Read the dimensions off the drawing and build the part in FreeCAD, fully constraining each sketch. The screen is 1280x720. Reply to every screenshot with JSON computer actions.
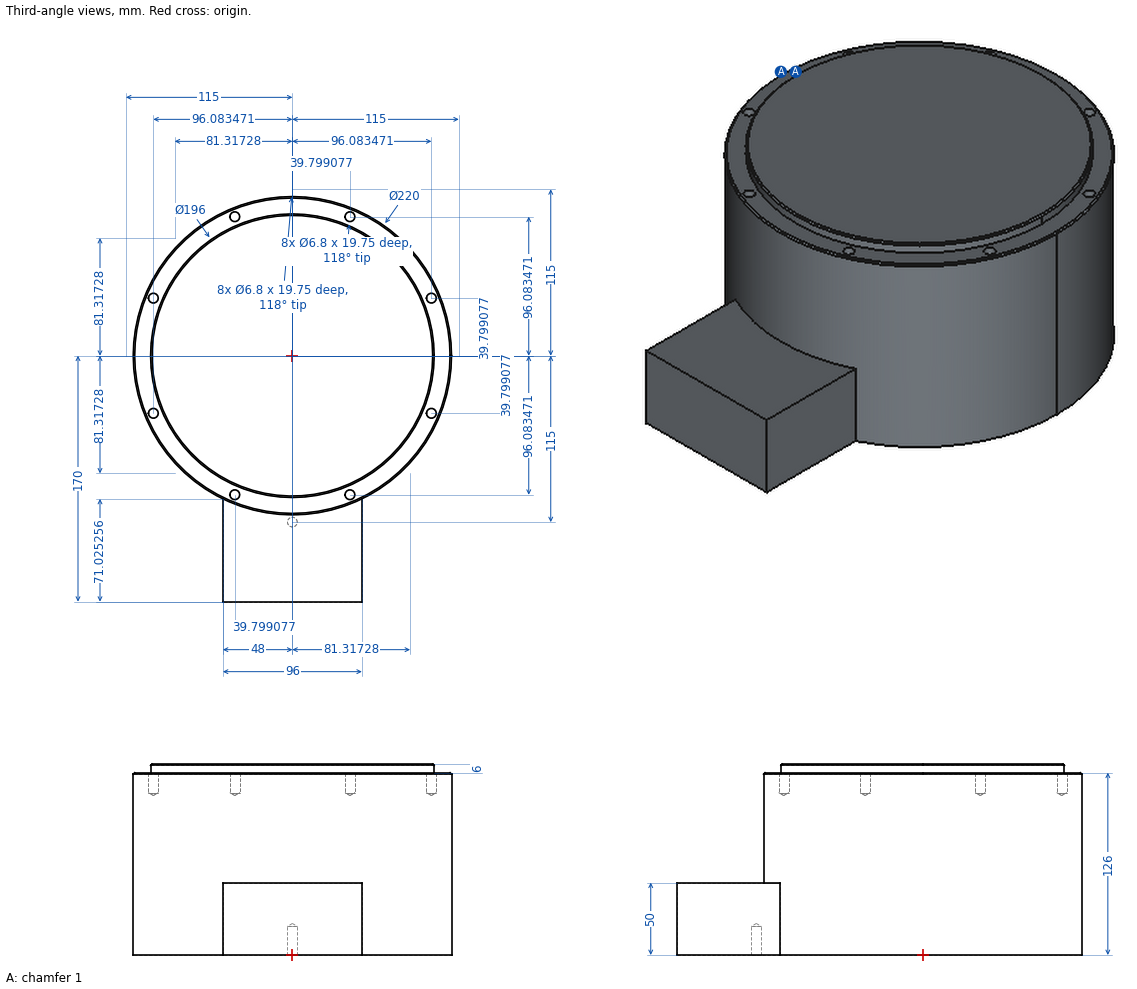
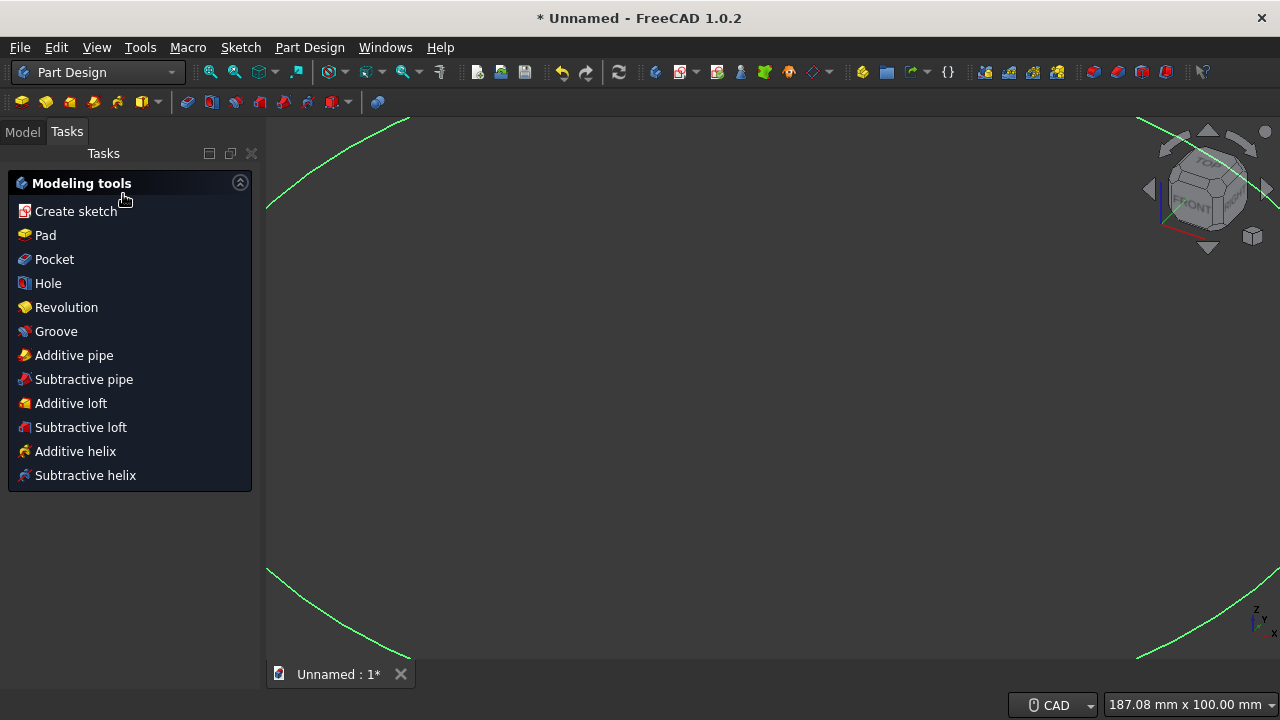
{"action": "left_click", "coordinate": [22, 102]}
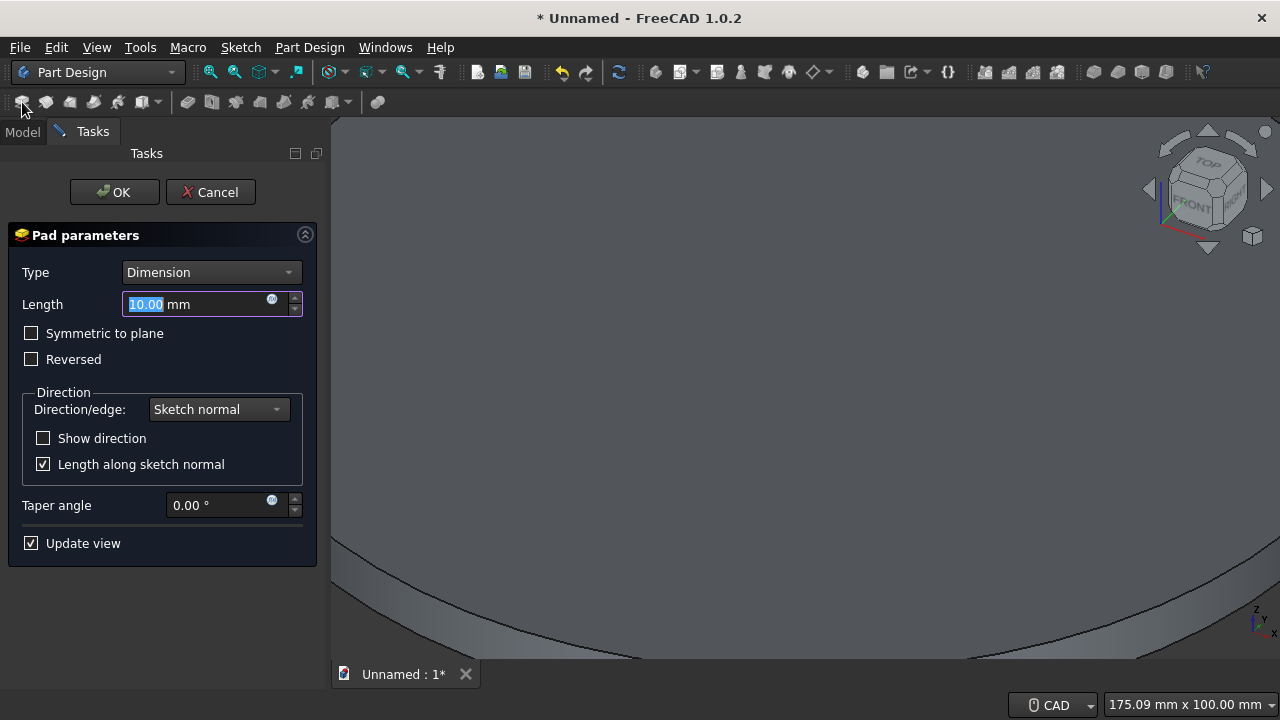
{"action": "type", "text": "126"}
{"action": "key", "text": "Tab"}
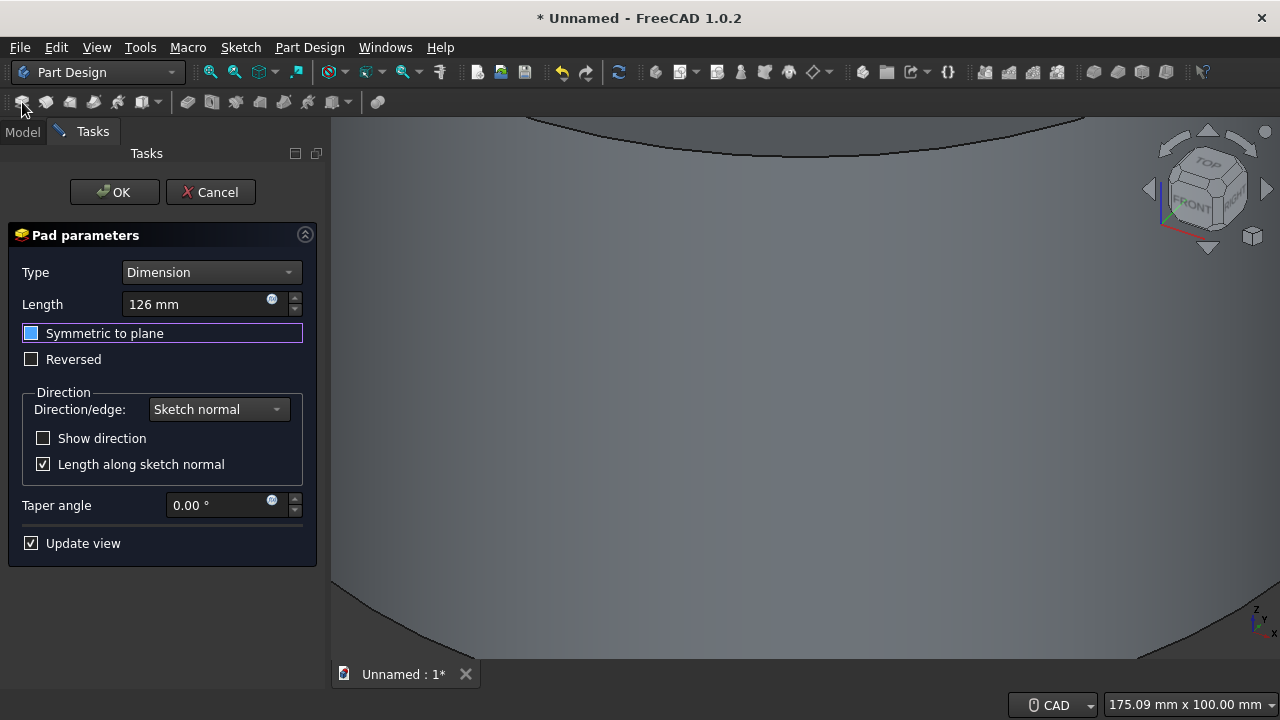
{"action": "left_click", "coordinate": [115, 192]}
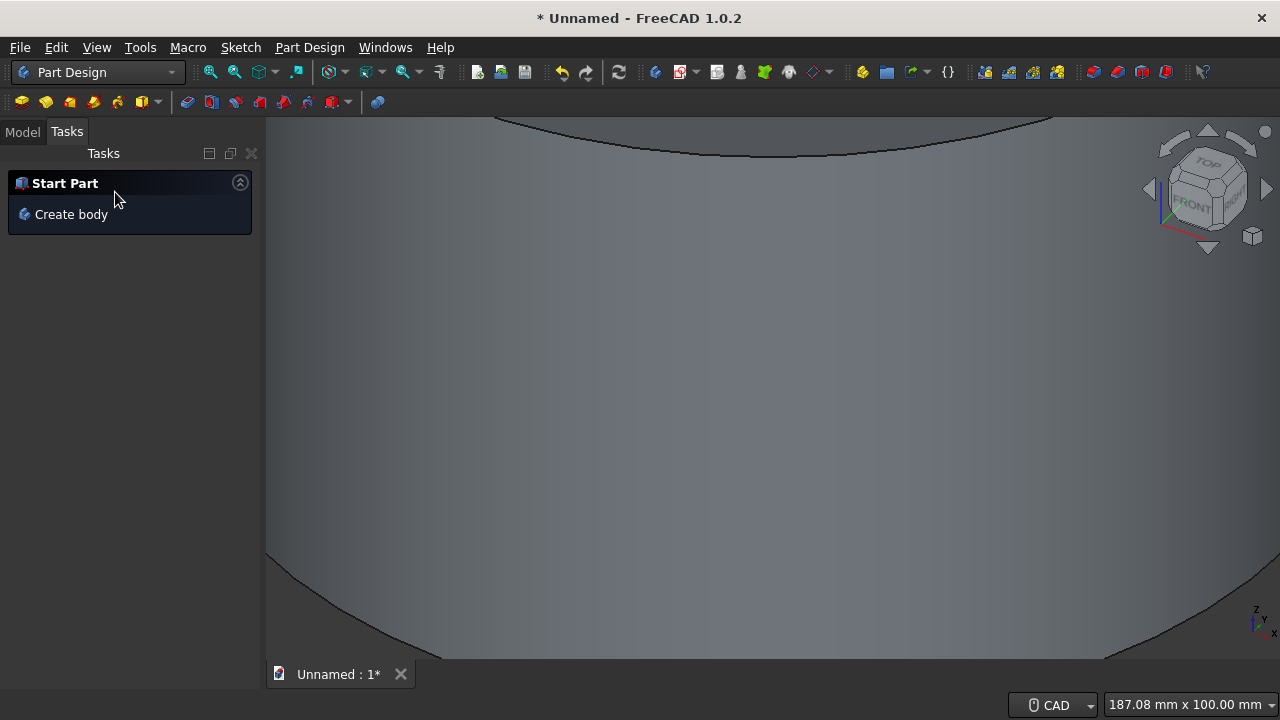
{"action": "left_click", "coordinate": [212, 72]}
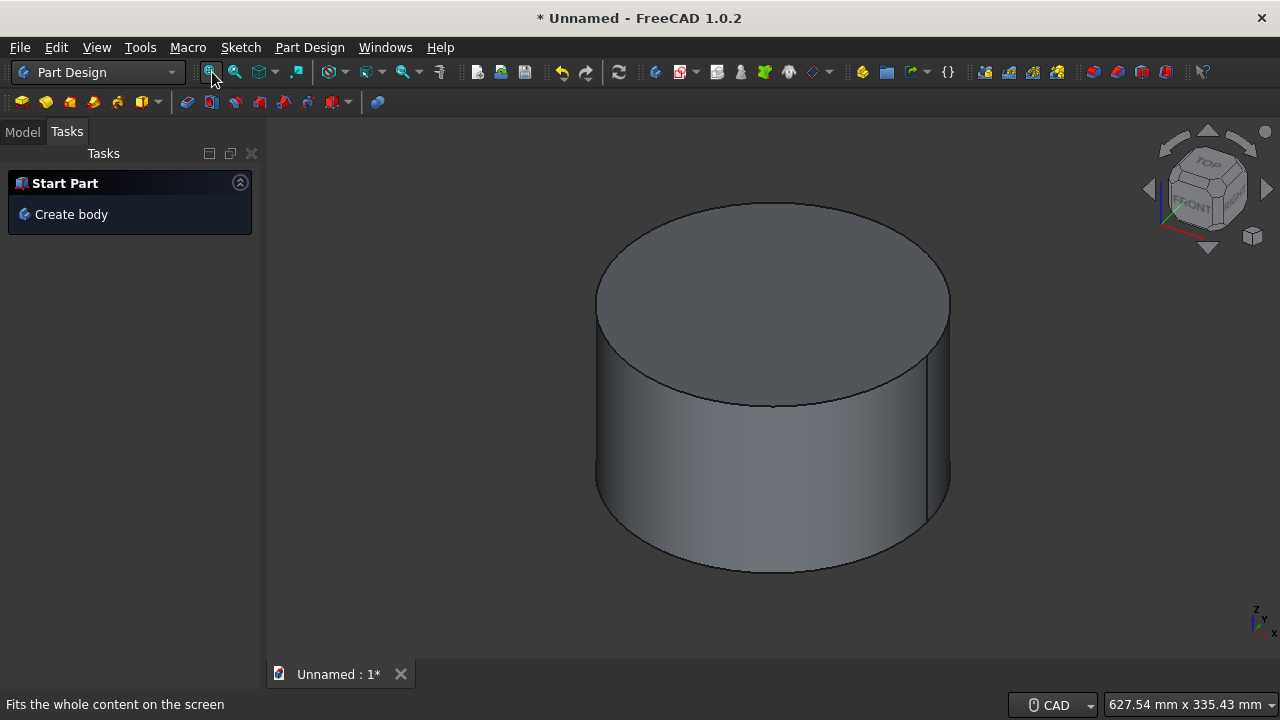
{"action": "left_click", "coordinate": [773, 304]}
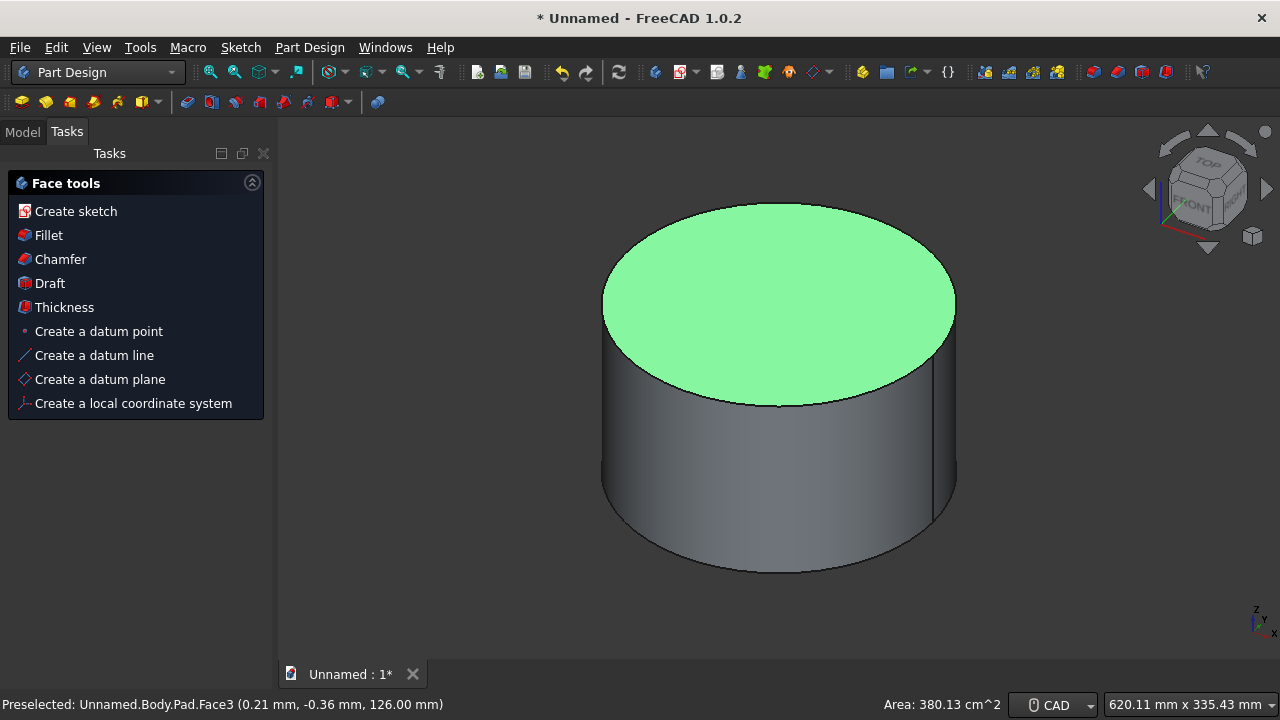
{"action": "left_click", "coordinate": [680, 72]}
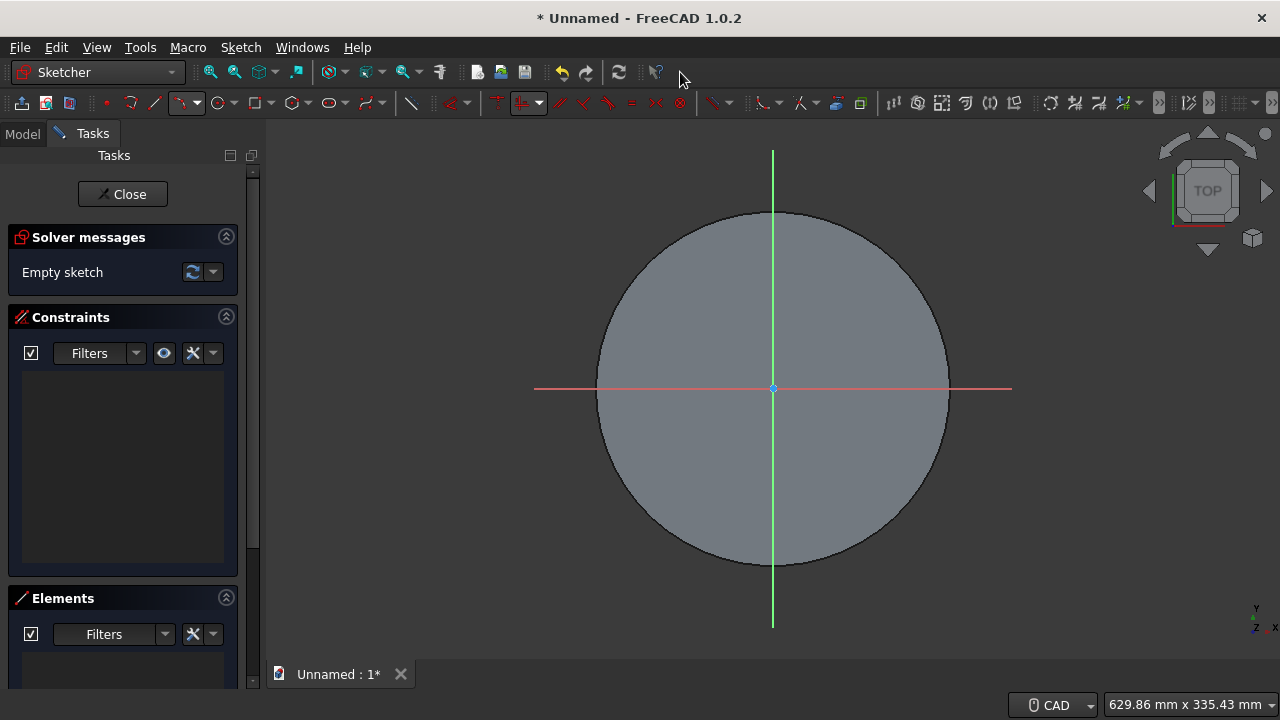
{"action": "left_click", "coordinate": [218, 104]}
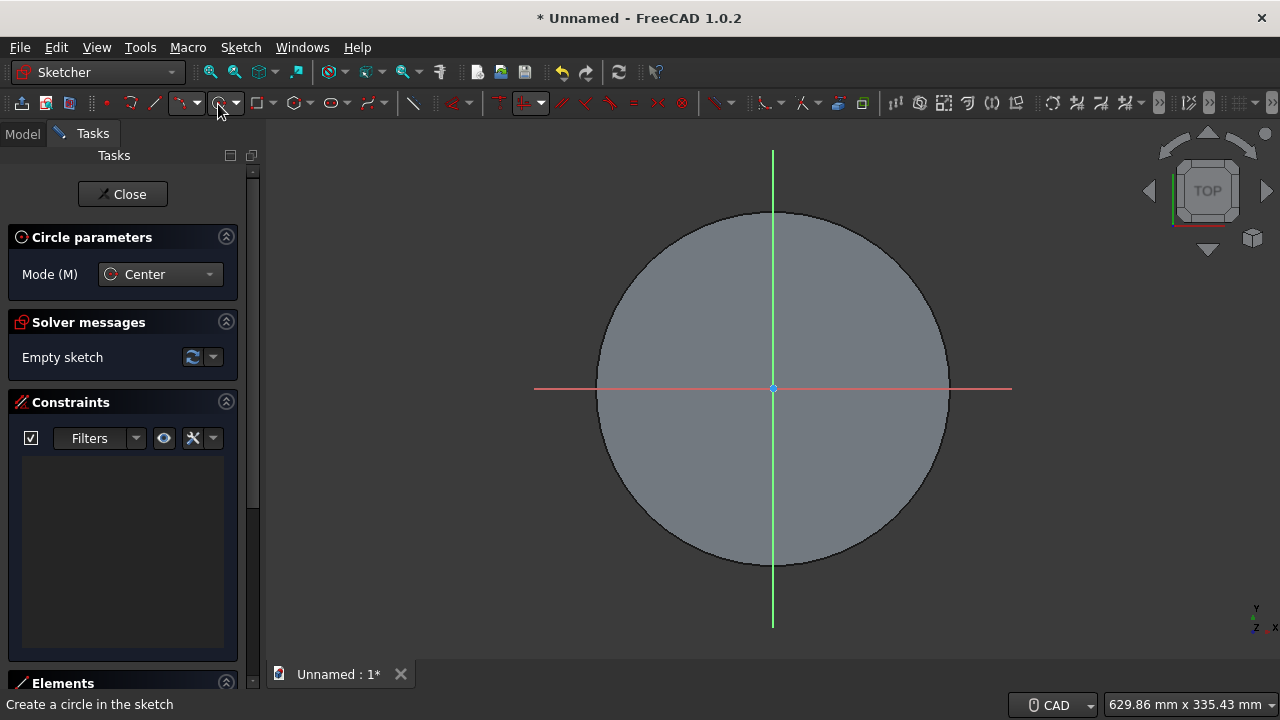
{"action": "left_click", "coordinate": [773, 389]}
{"action": "left_click", "coordinate": [885, 277]}
{"action": "key", "text": "Escape"}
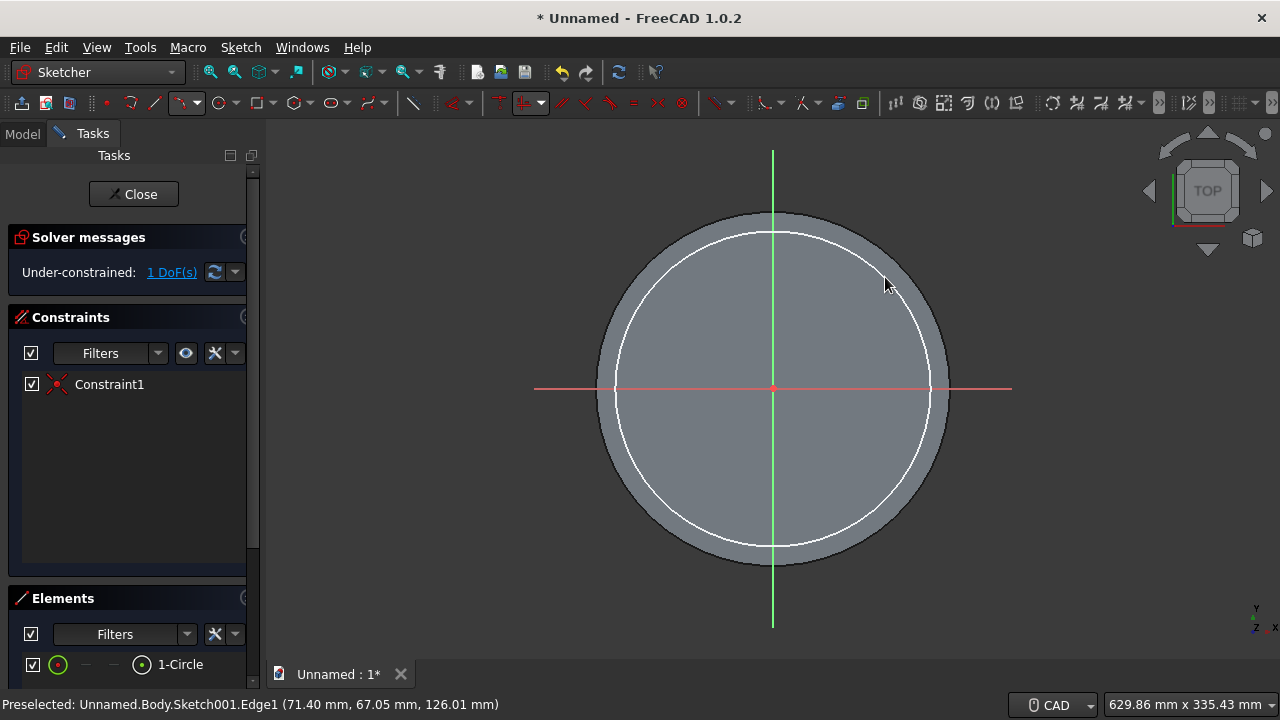
{"action": "left_click", "coordinate": [452, 104]}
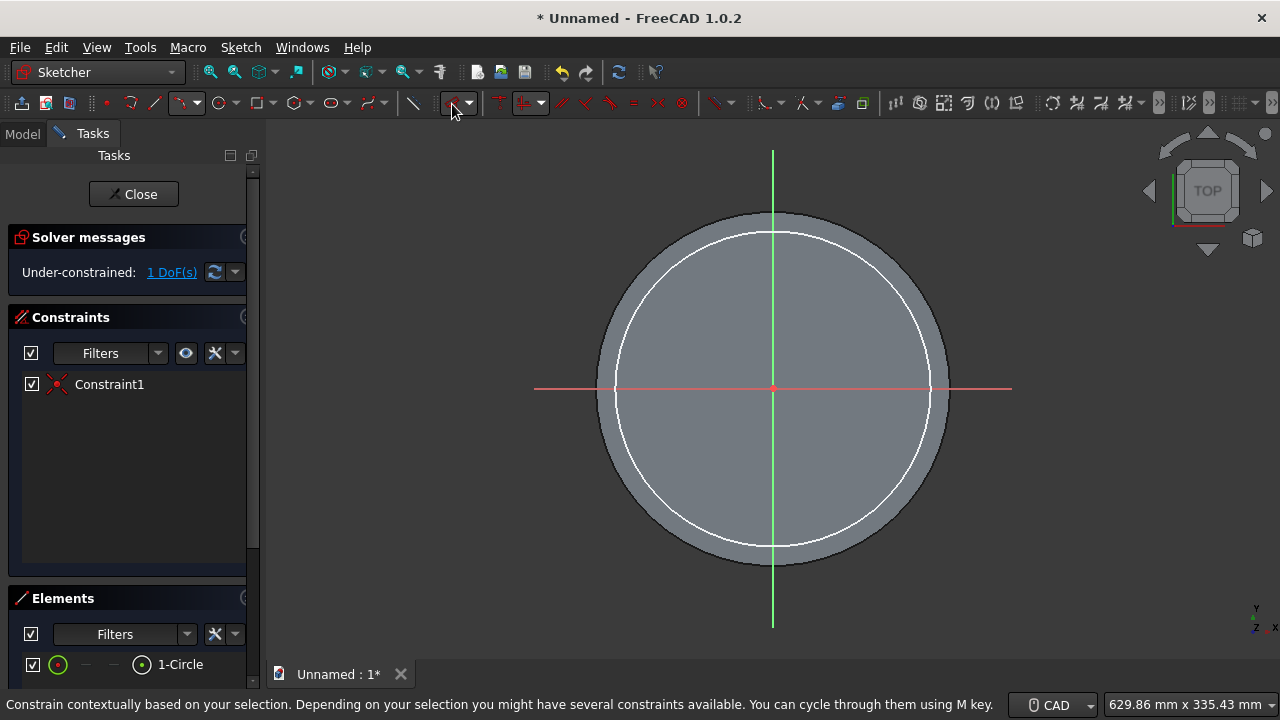
{"action": "left_click", "coordinate": [884, 277]}
{"action": "left_click", "coordinate": [907, 254]}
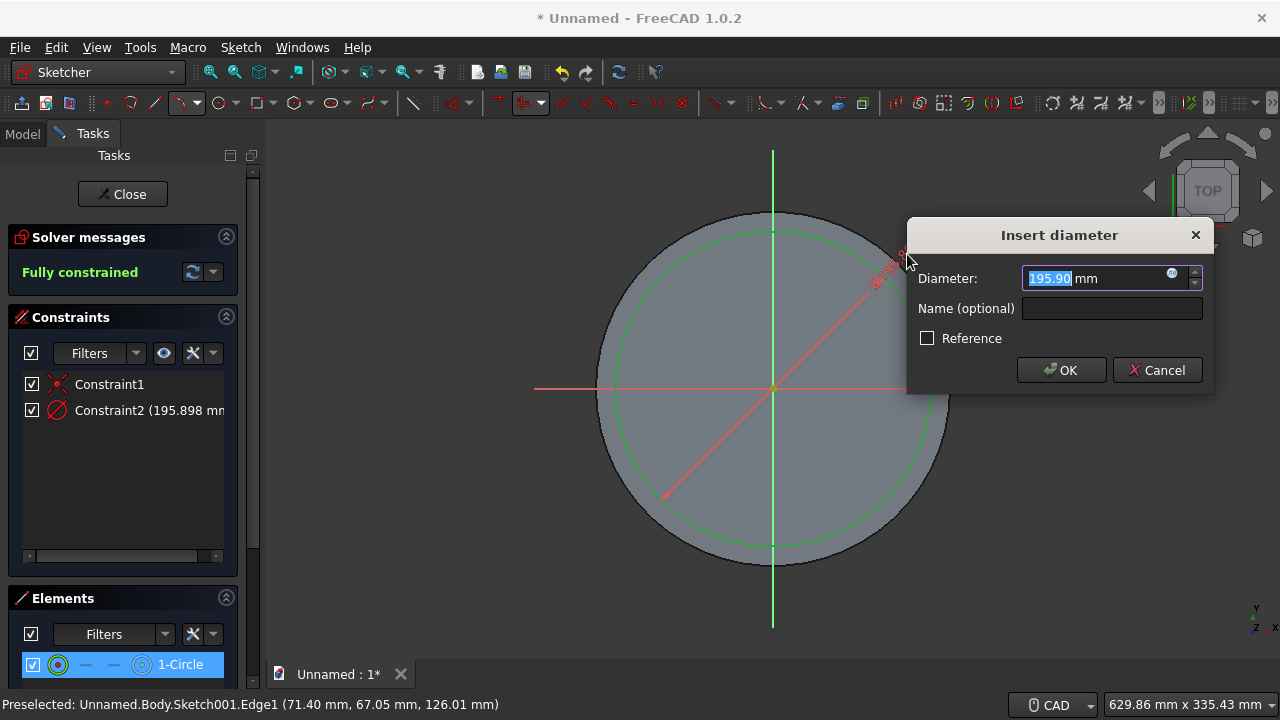
{"action": "type", "text": "196"}
{"action": "key", "text": "Return"}
{"action": "key", "text": "Escape"}